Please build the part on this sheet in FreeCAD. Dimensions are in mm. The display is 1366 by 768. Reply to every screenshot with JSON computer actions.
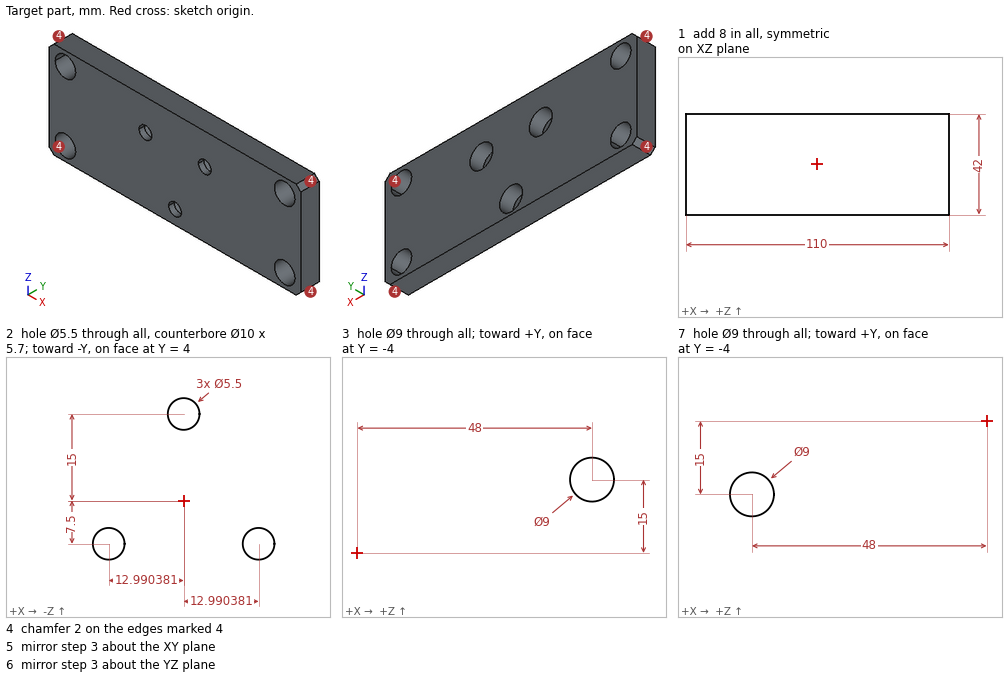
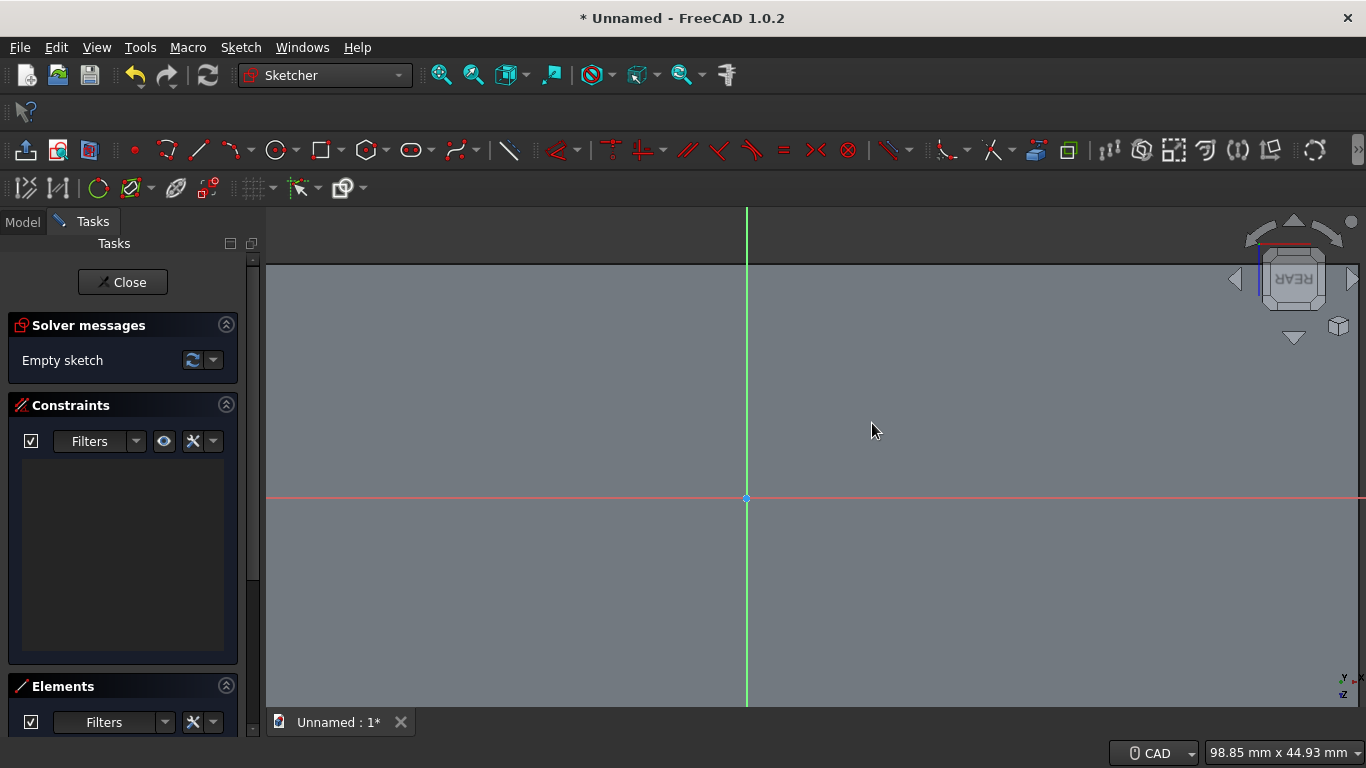
{"action": "left_click", "coordinate": [276, 150]}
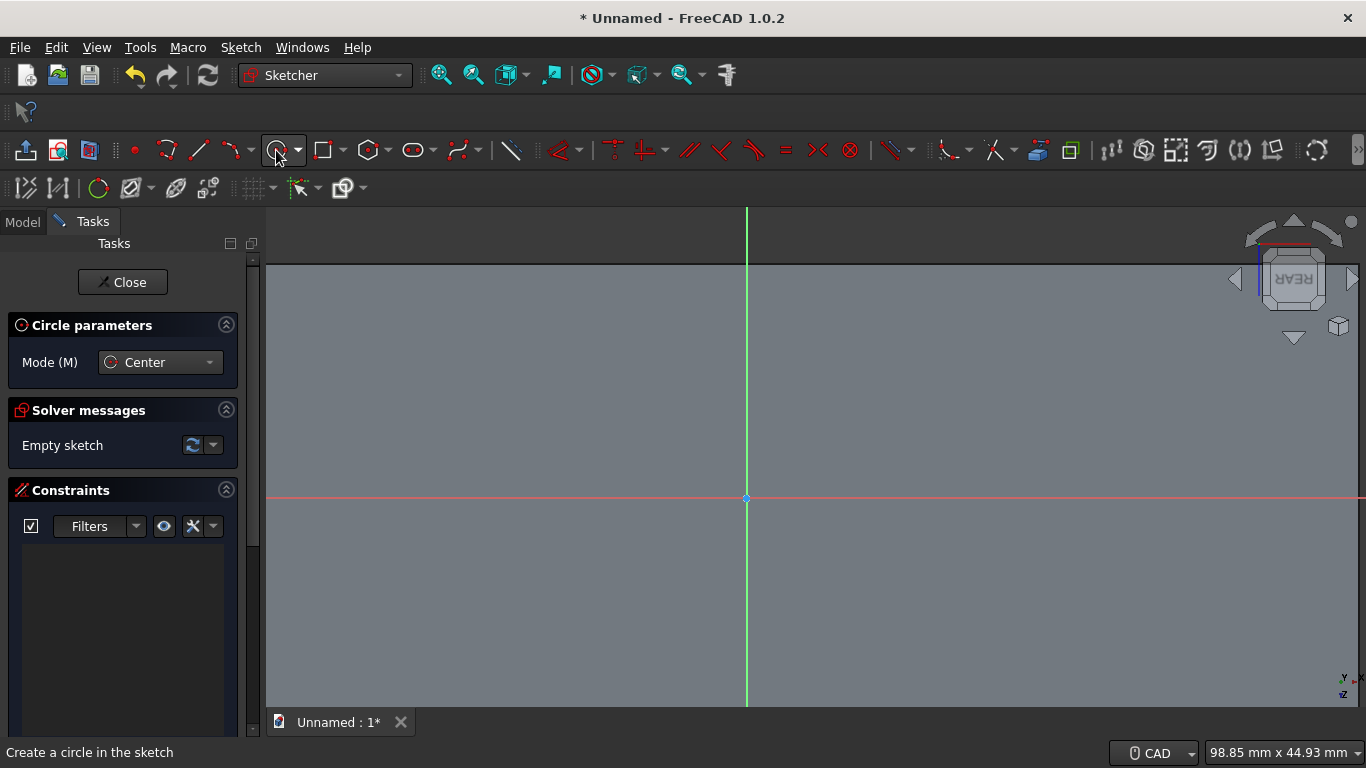
{"action": "left_click", "coordinate": [747, 331]}
{"action": "left_click", "coordinate": [768, 310]}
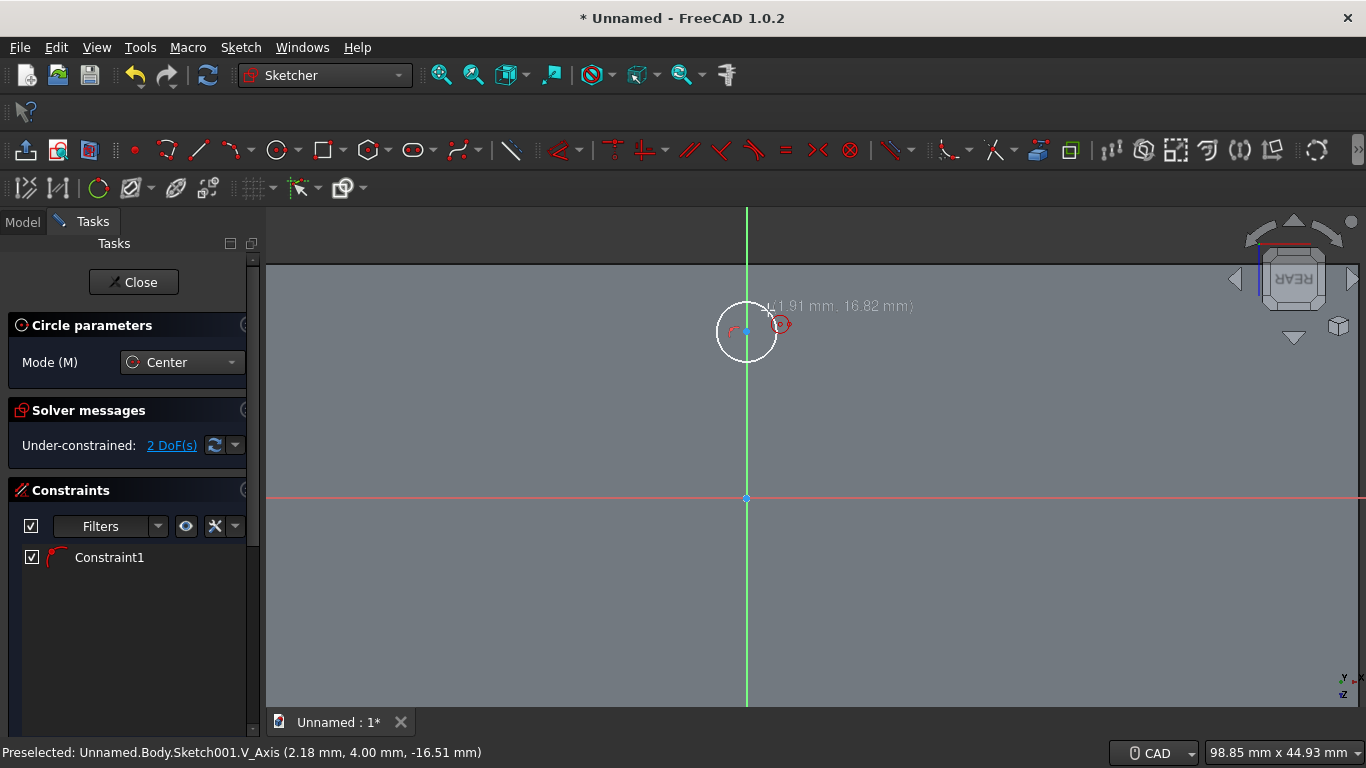
{"action": "left_click", "coordinate": [602, 582]}
{"action": "left_click", "coordinate": [624, 560]}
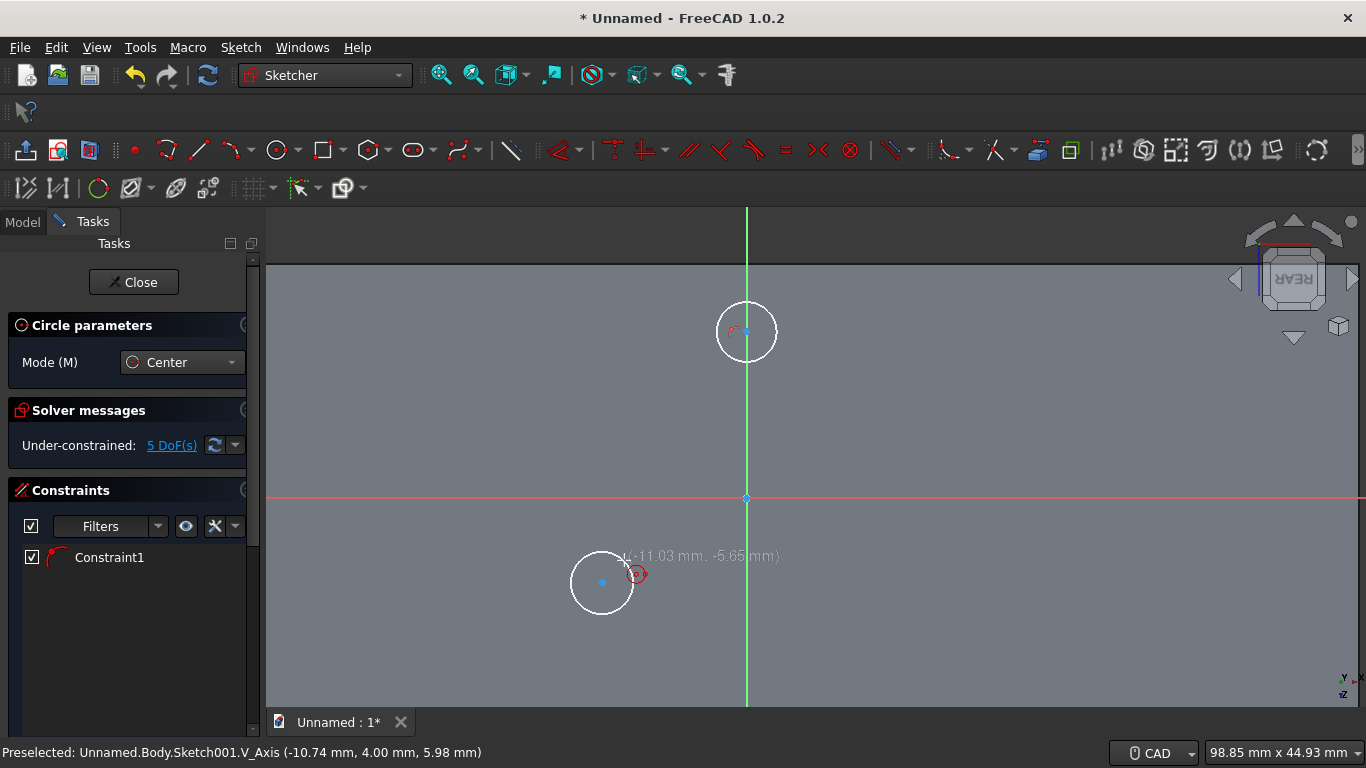
{"action": "left_click", "coordinate": [891, 582]}
{"action": "left_click", "coordinate": [913, 560]}
{"action": "key", "text": "Escape"}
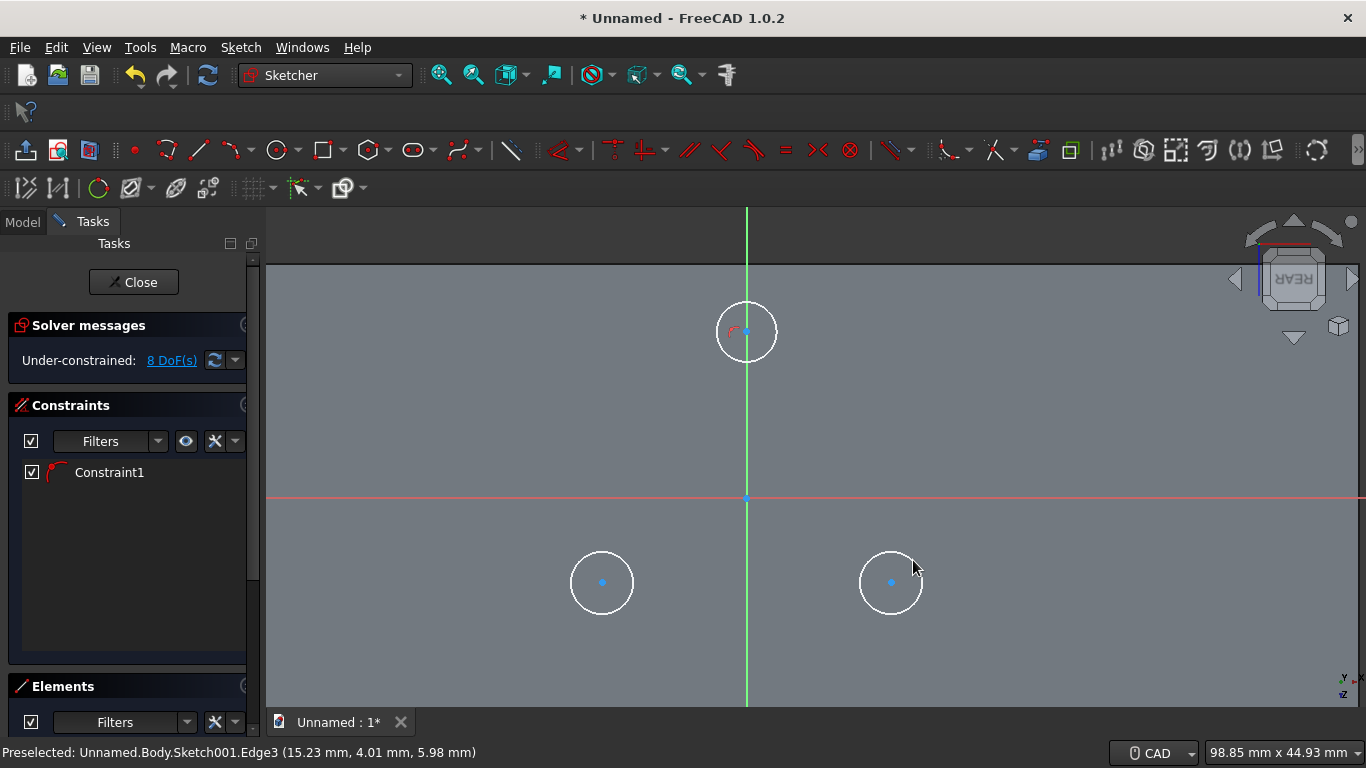
{"action": "left_click", "coordinate": [768, 311]}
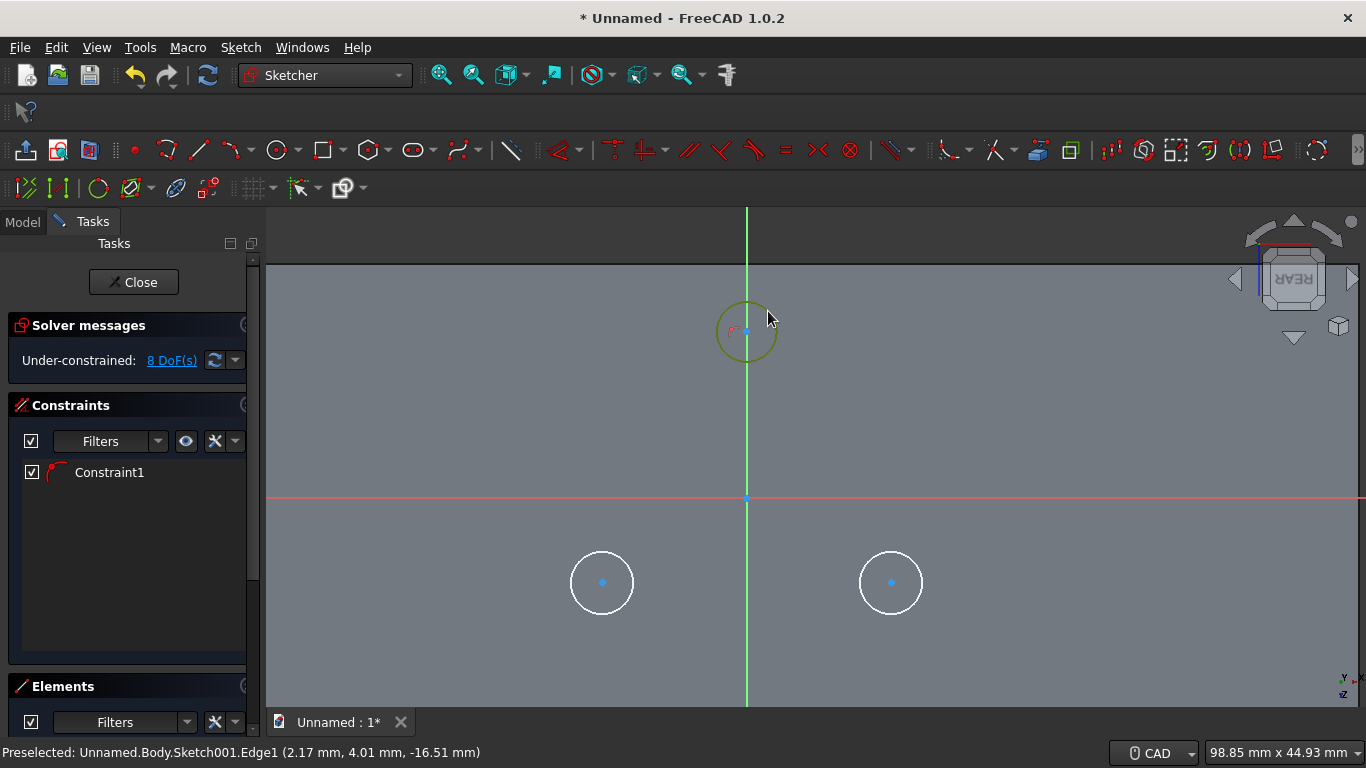
{"action": "left_click", "coordinate": [624, 561]}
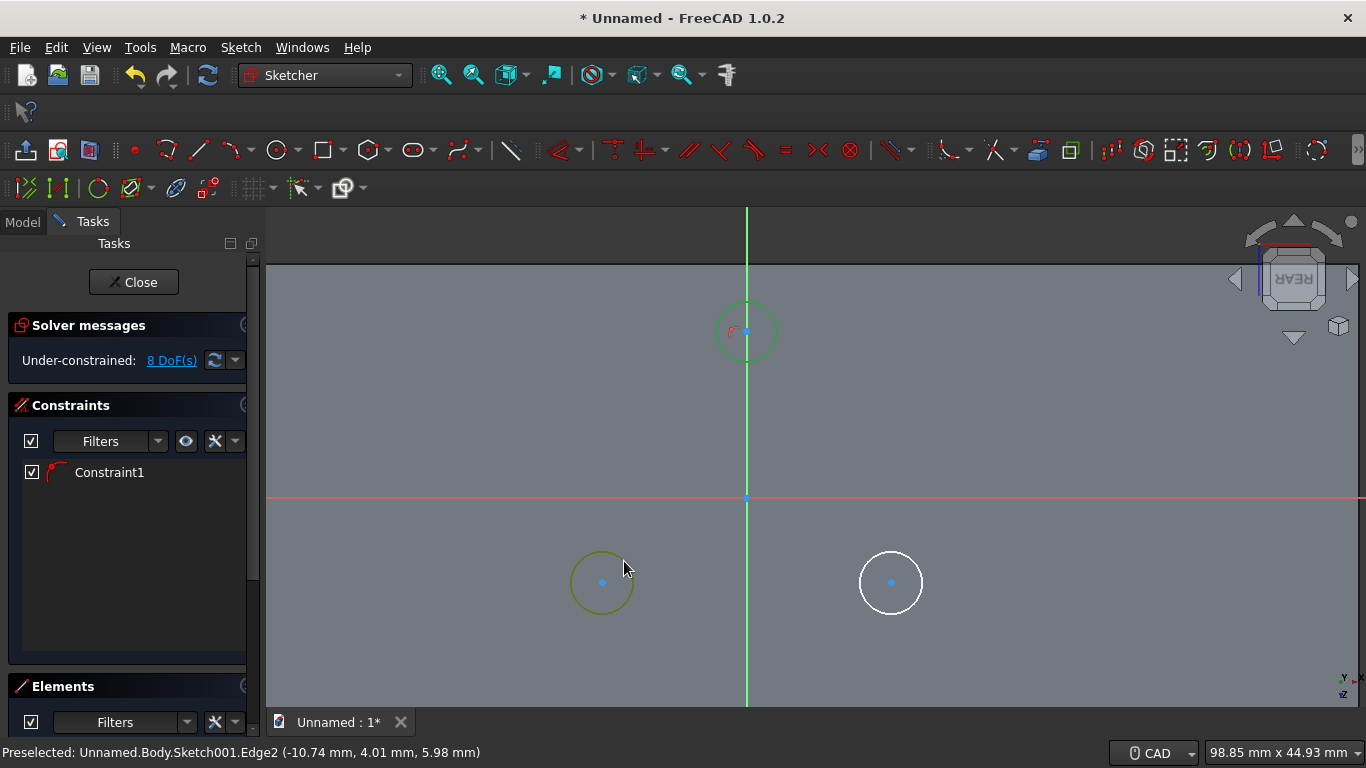
{"action": "left_click", "coordinate": [913, 561]}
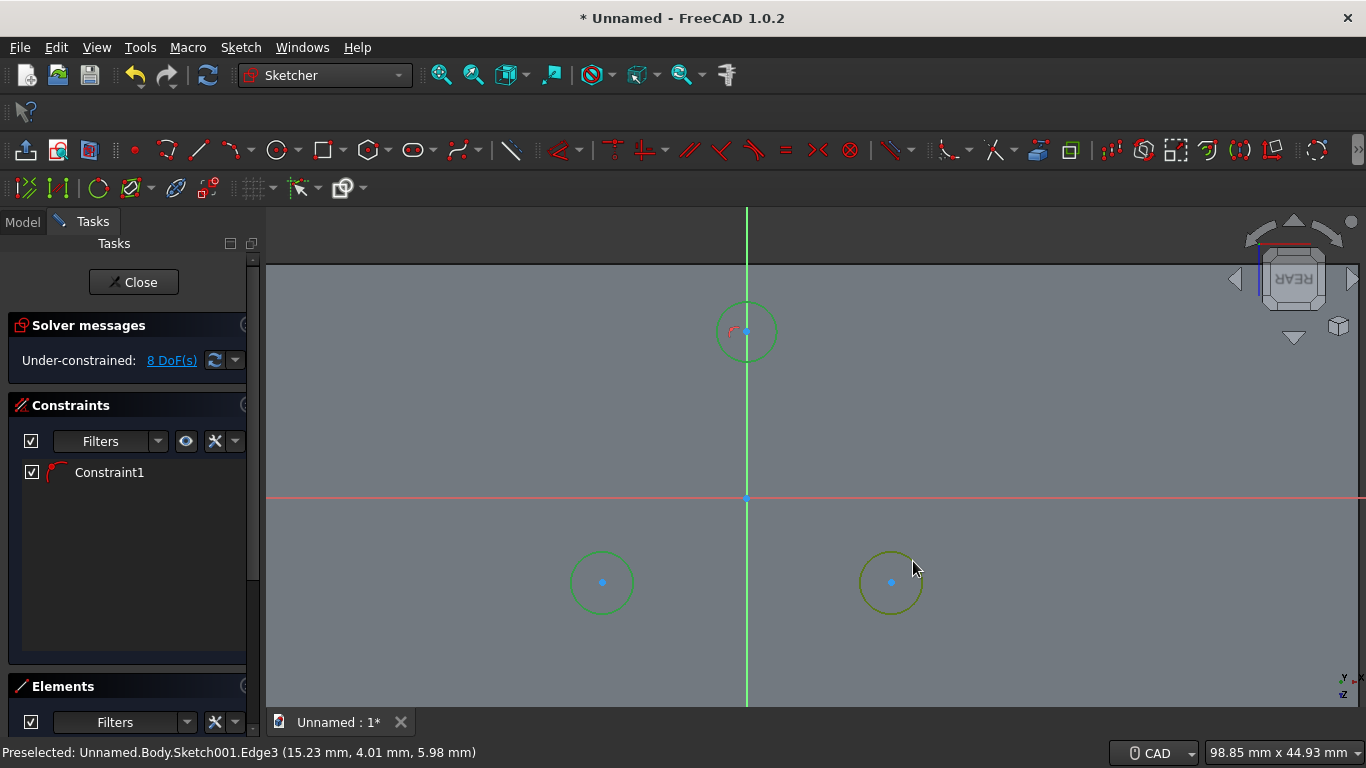
{"action": "left_click", "coordinate": [786, 150]}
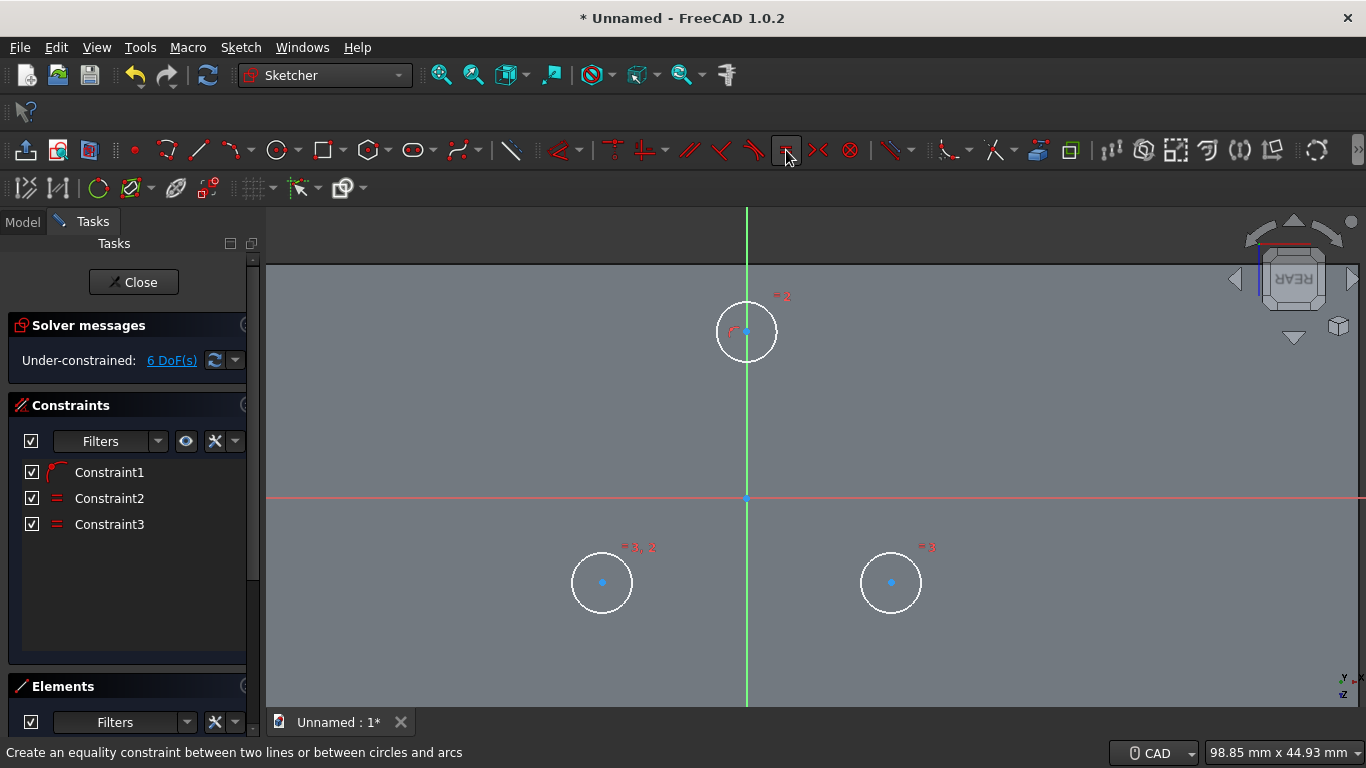
{"action": "left_click", "coordinate": [602, 583]}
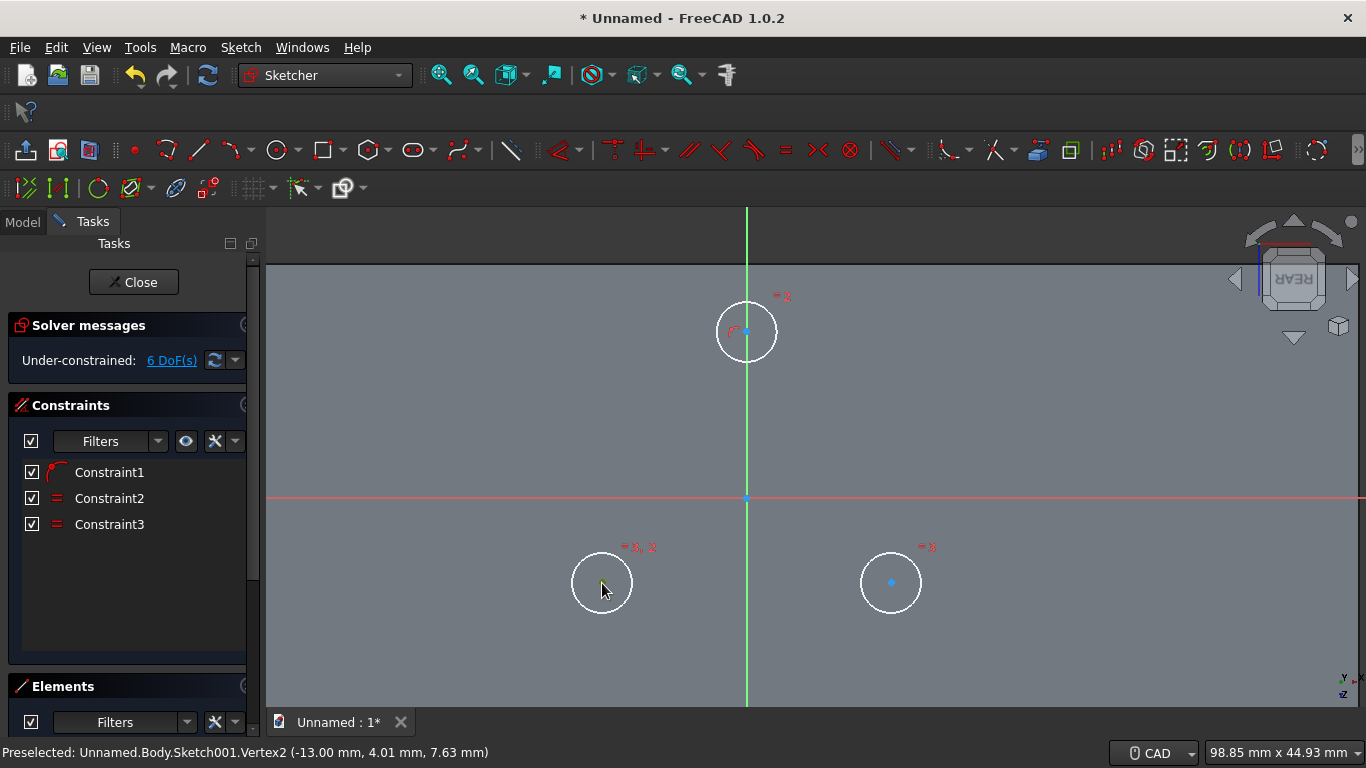
{"action": "left_click", "coordinate": [891, 583]}